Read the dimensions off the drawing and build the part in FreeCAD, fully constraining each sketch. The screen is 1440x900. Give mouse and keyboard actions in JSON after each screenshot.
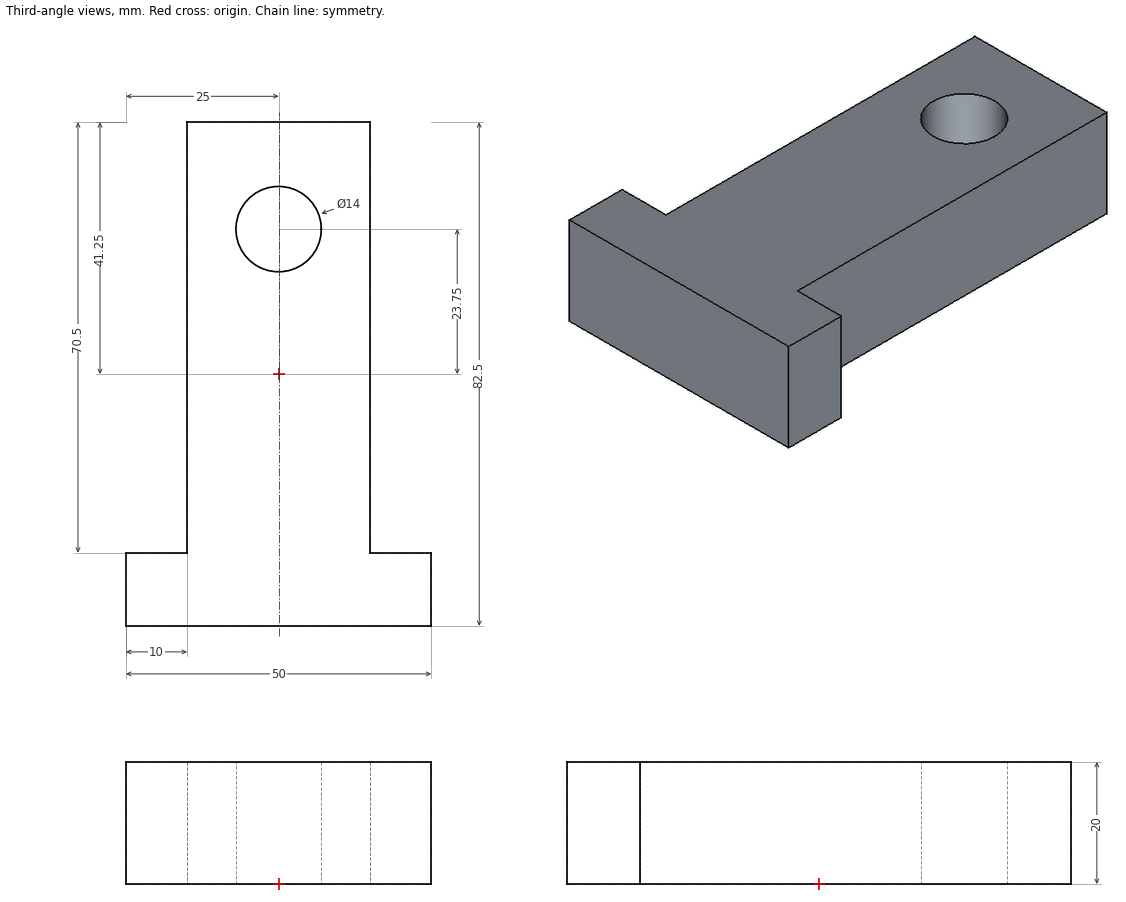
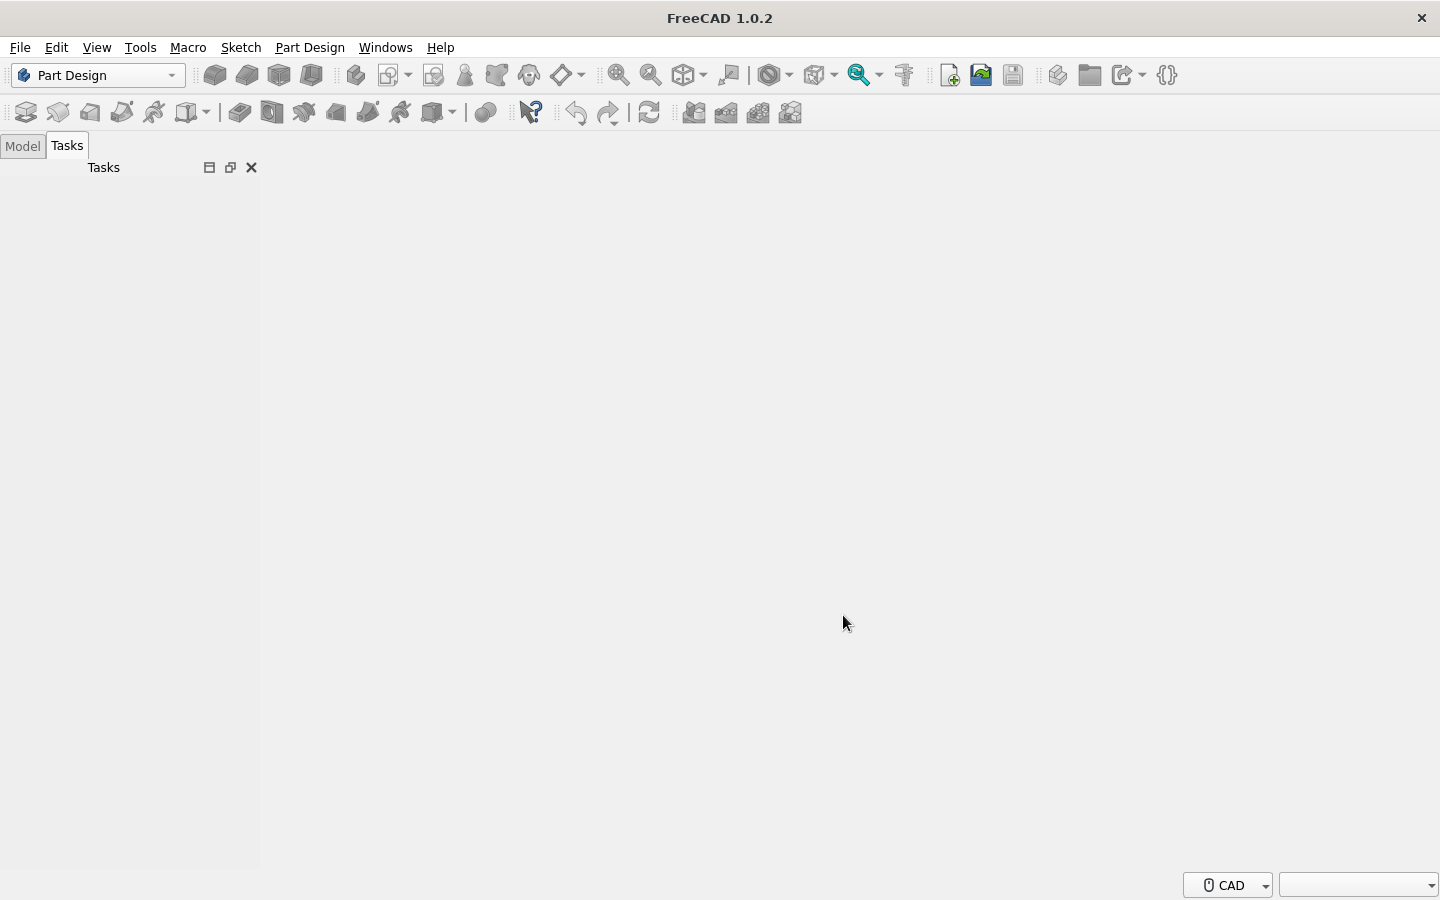
{"action": "left_click", "coordinate": [950, 76]}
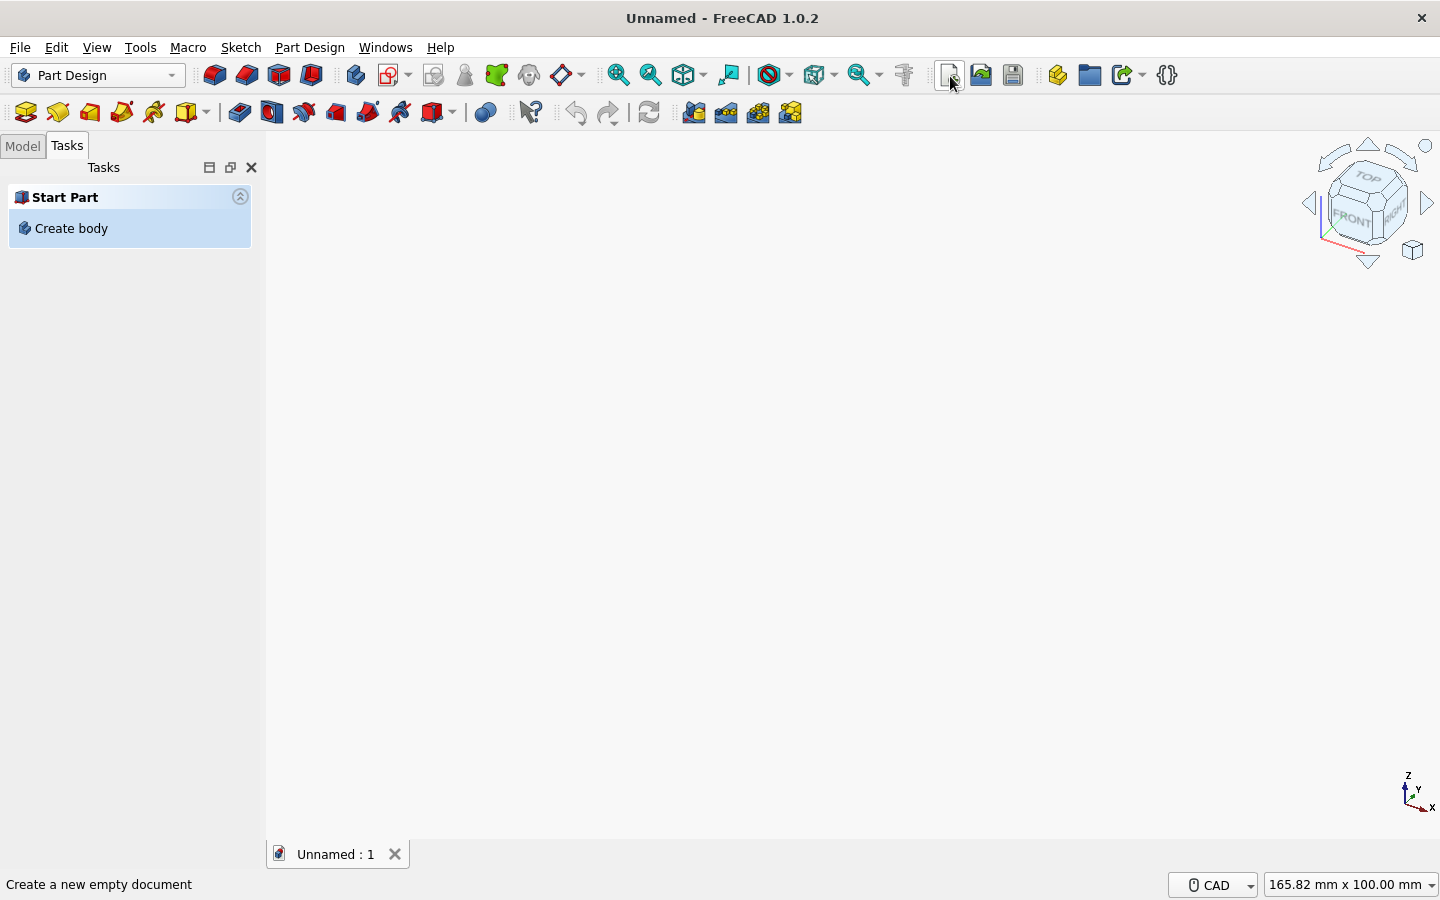
{"action": "left_click", "coordinate": [388, 76]}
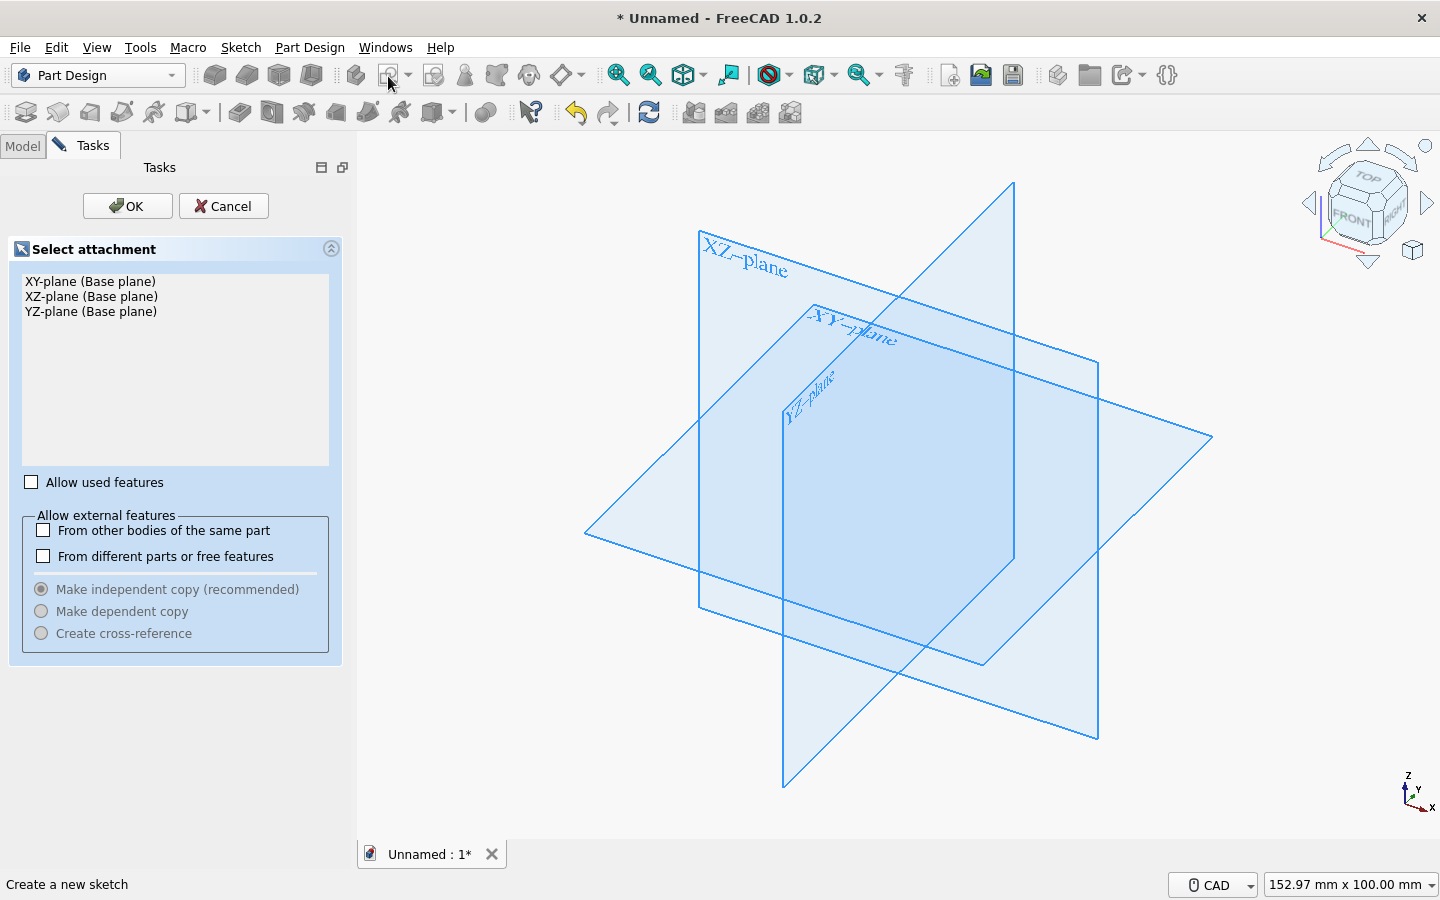
{"action": "left_click", "coordinate": [82, 282]}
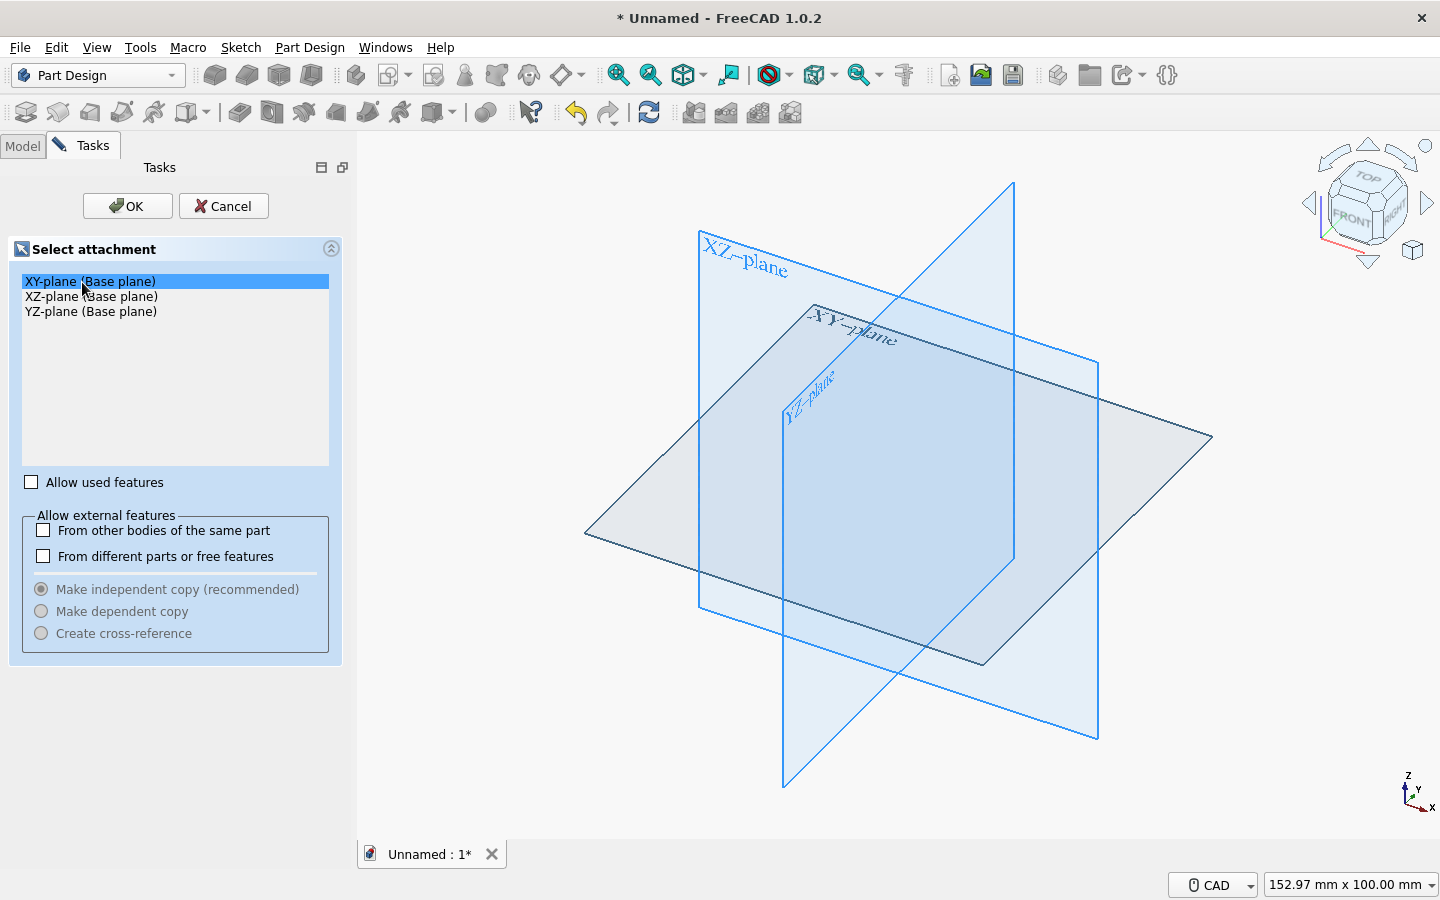
{"action": "left_click", "coordinate": [128, 206]}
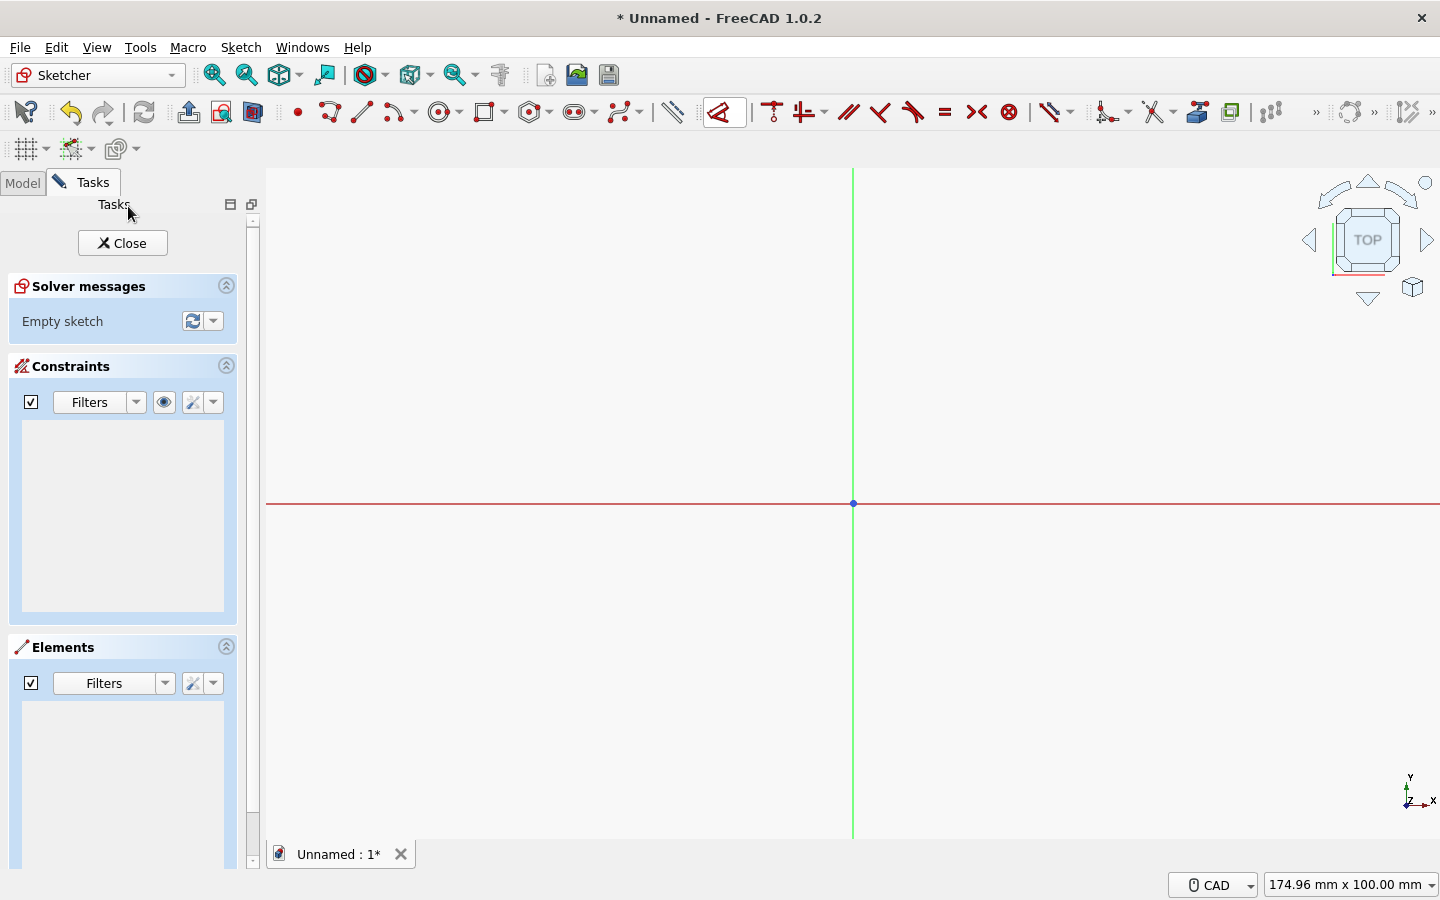
{"action": "key", "text": "g v"}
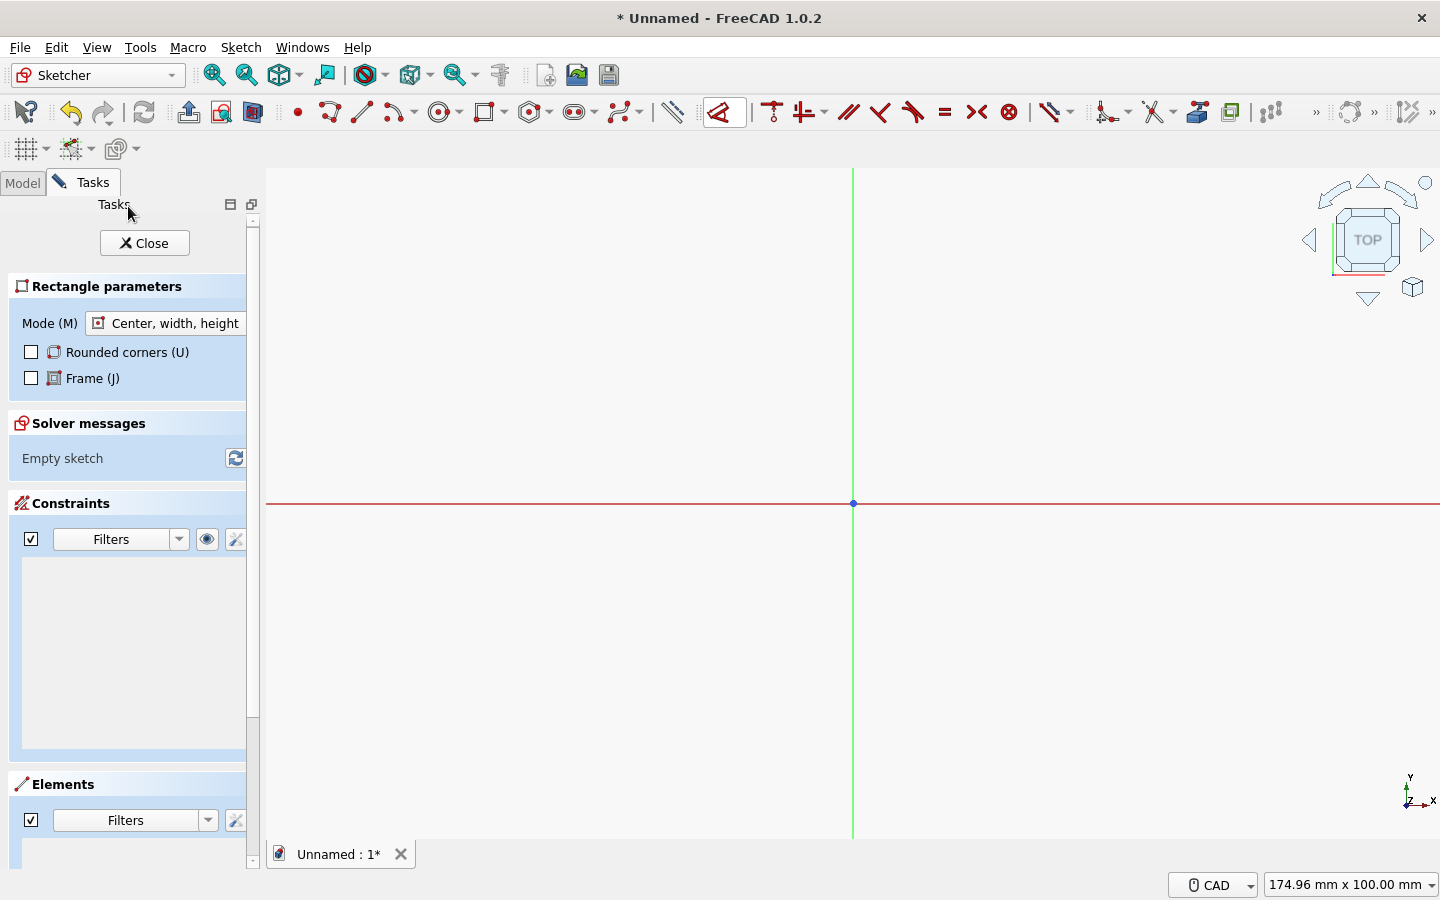
{"action": "left_click", "coordinate": [853, 504]}
{"action": "left_click", "coordinate": [1021, 227]}
{"action": "key", "text": "Escape"}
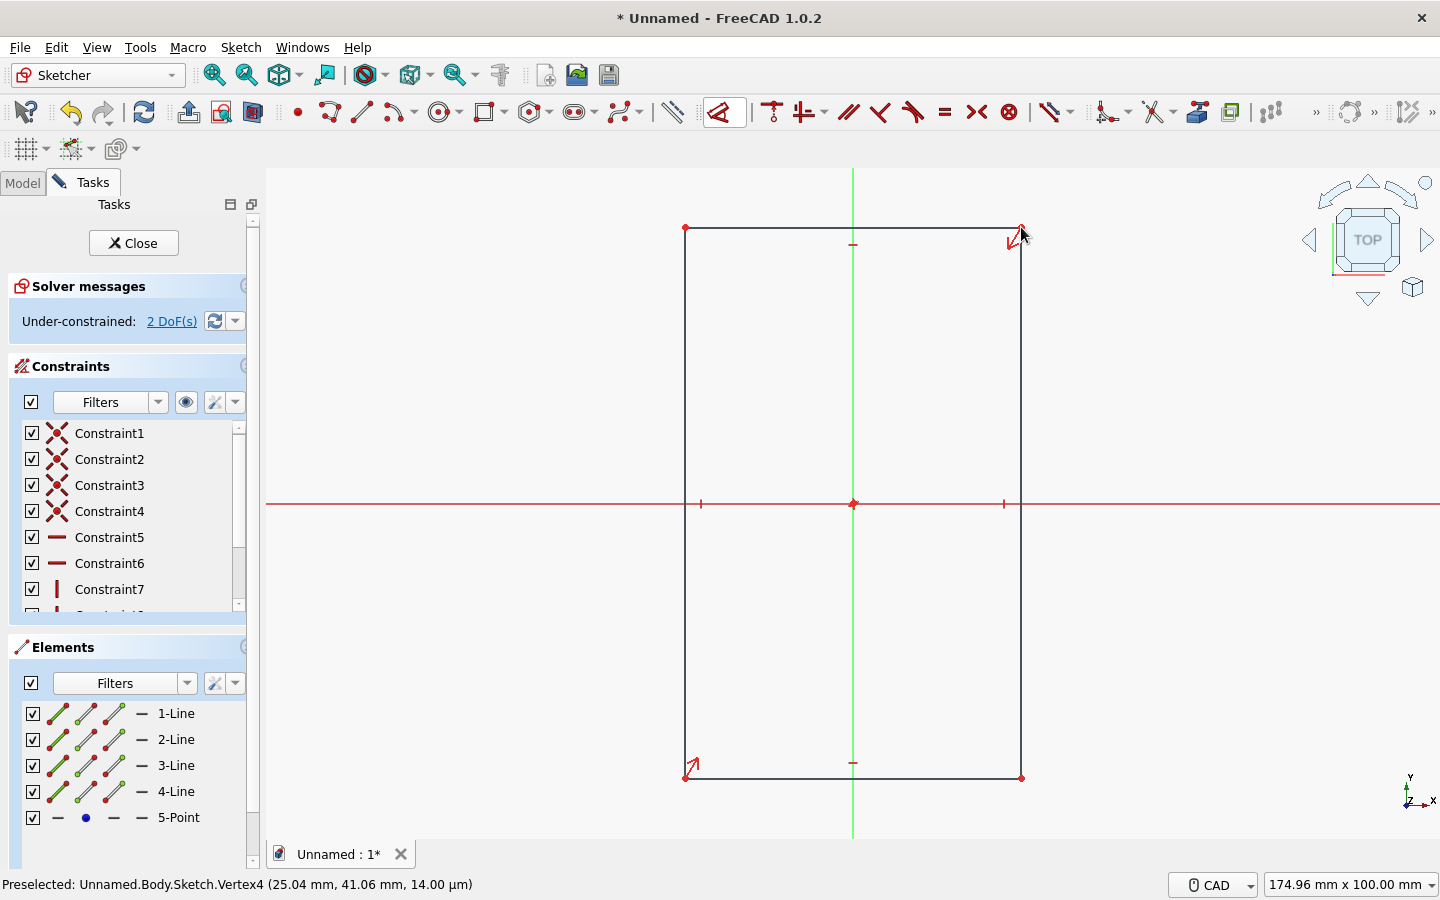
{"action": "left_click", "coordinate": [718, 112]}